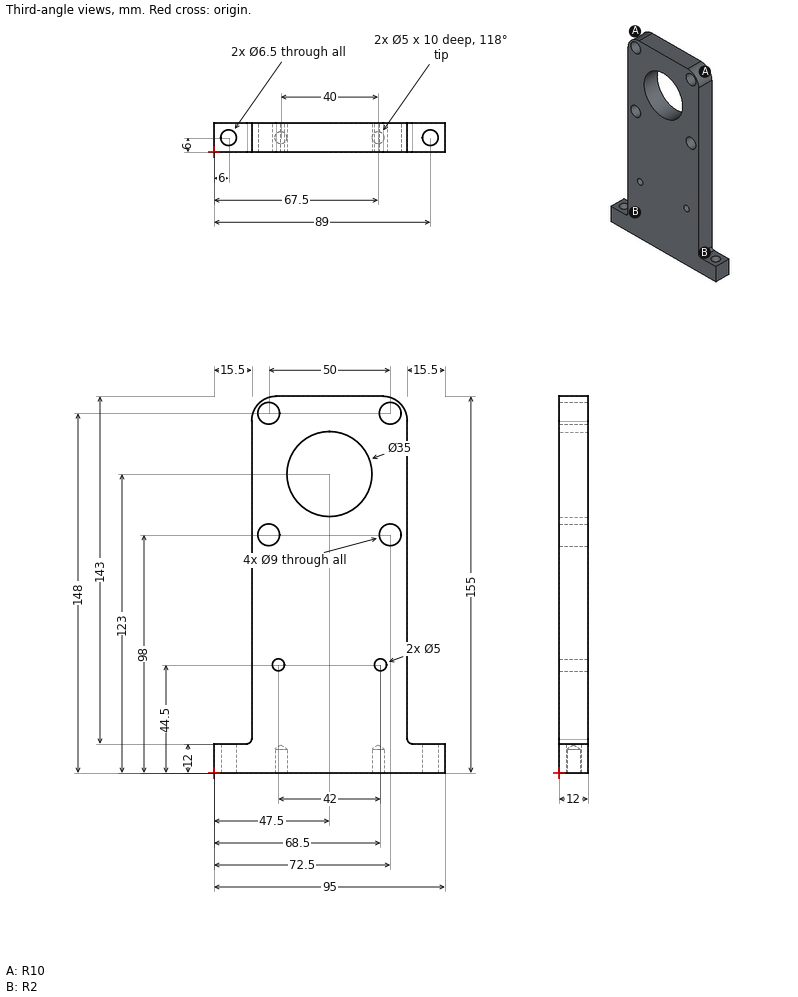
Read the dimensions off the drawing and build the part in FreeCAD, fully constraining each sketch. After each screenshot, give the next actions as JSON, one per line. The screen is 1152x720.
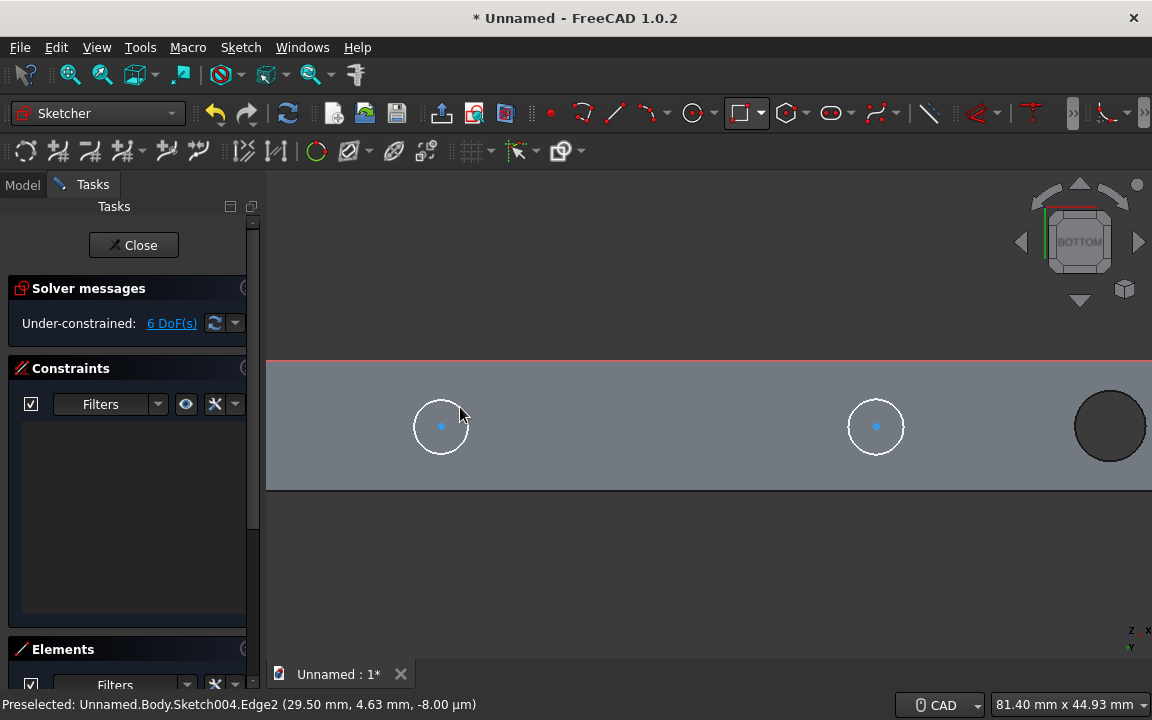
{"action": "left_click", "coordinate": [895, 407]}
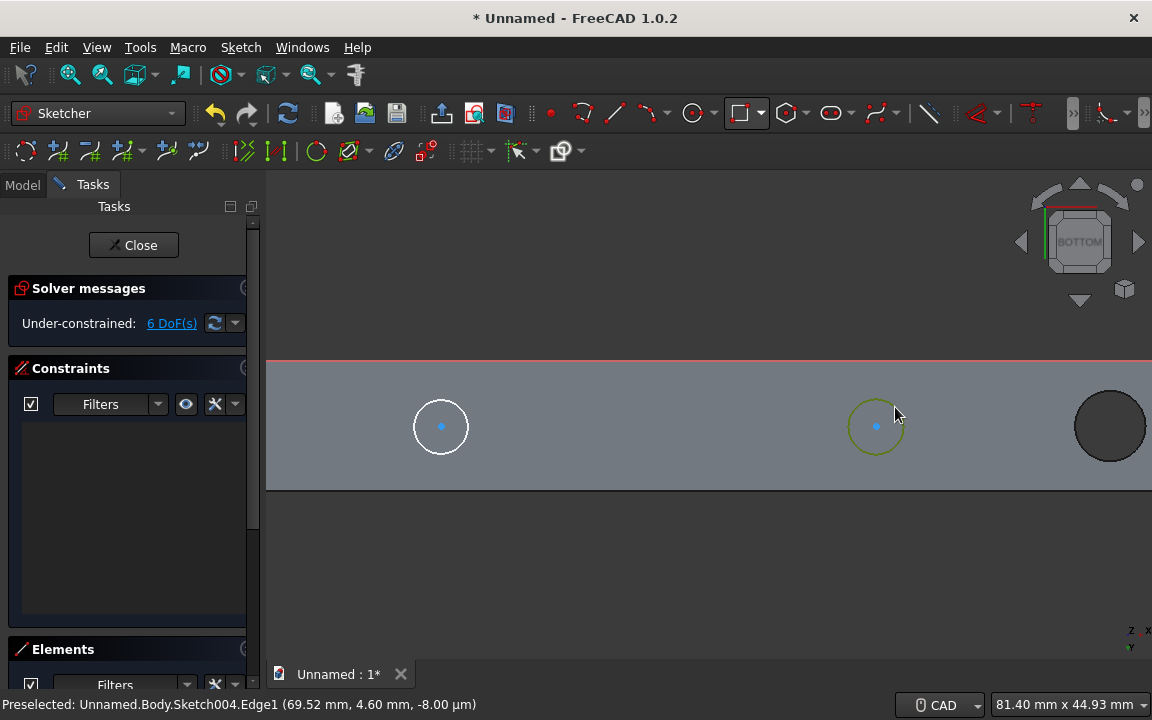
{"action": "left_click", "coordinate": [460, 408]}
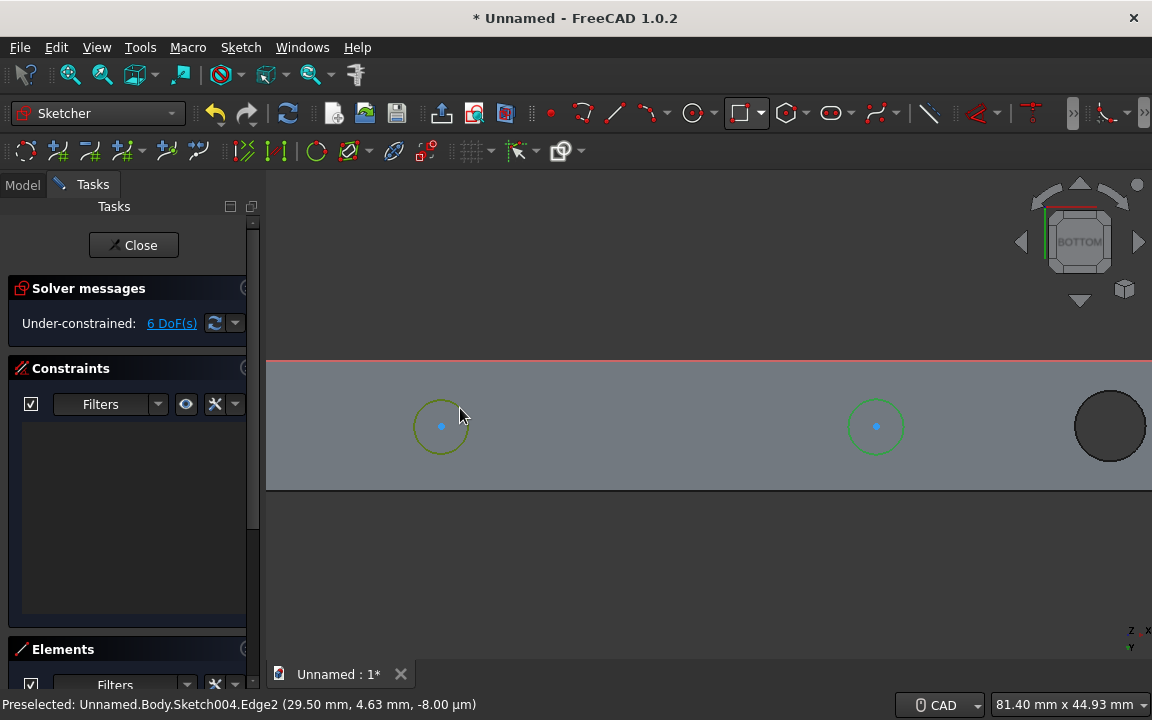
{"action": "key", "text": "e"}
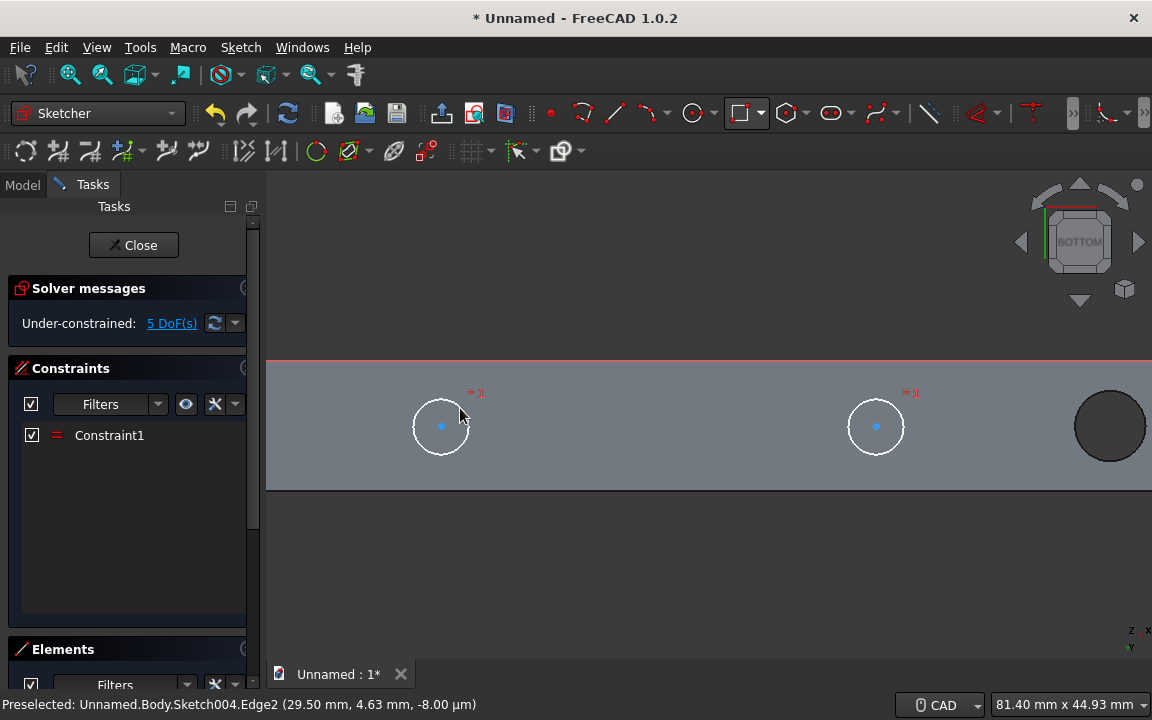
{"action": "left_click", "coordinate": [876, 427]}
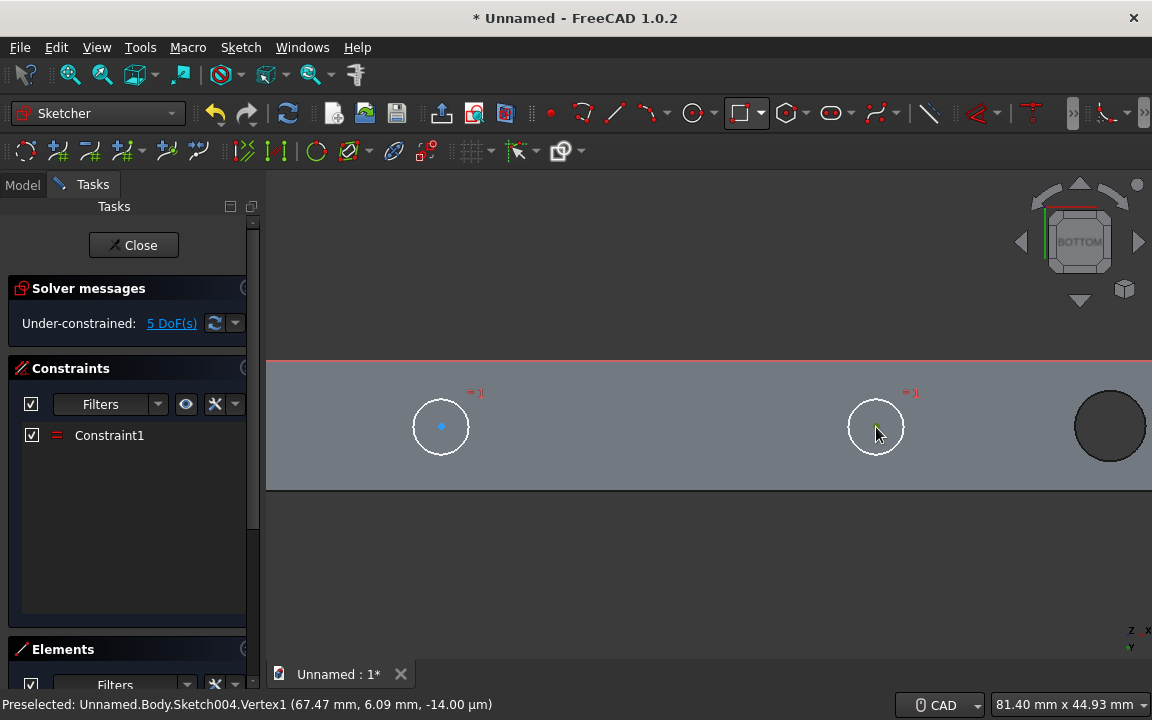
{"action": "left_click", "coordinate": [441, 427]}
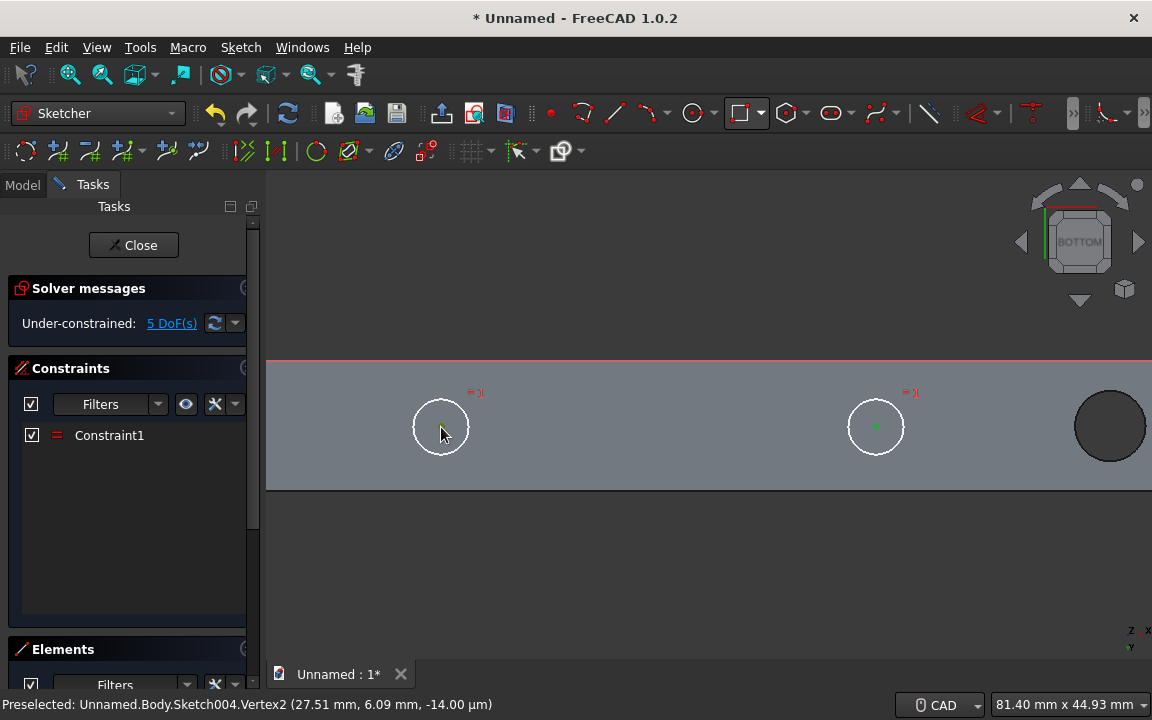
{"action": "key", "text": "h"}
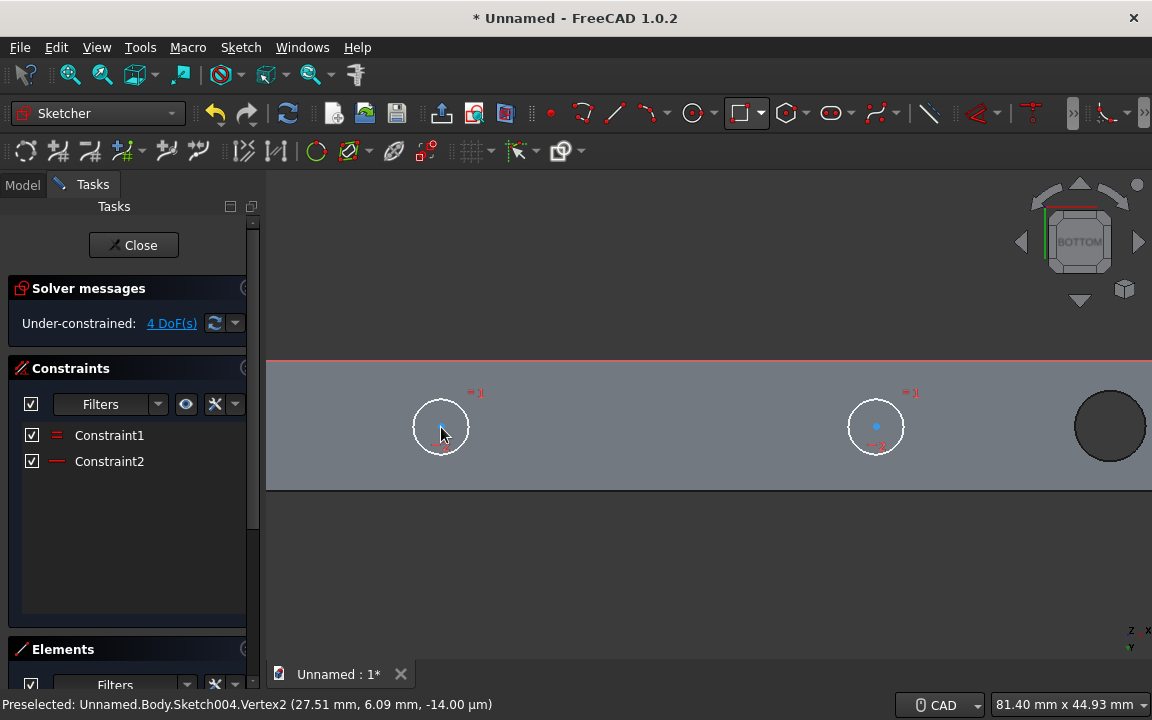
{"action": "left_click", "coordinate": [976, 114]}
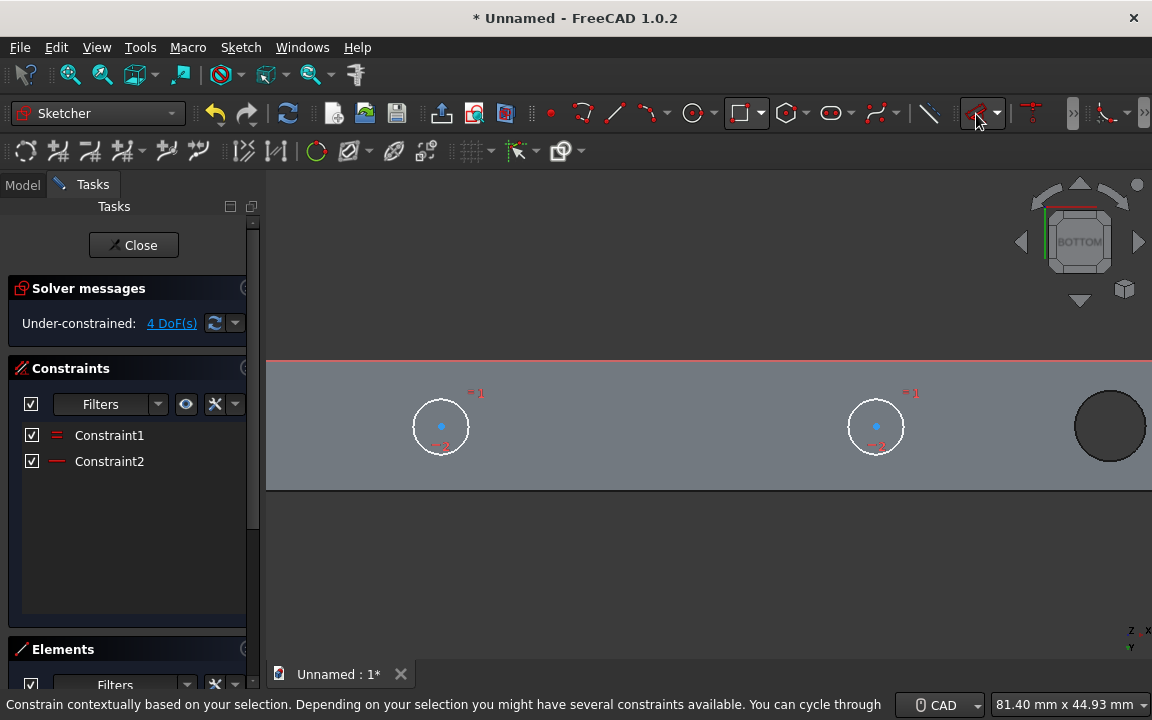
{"action": "left_click", "coordinate": [895, 407]}
{"action": "left_click", "coordinate": [917, 384]}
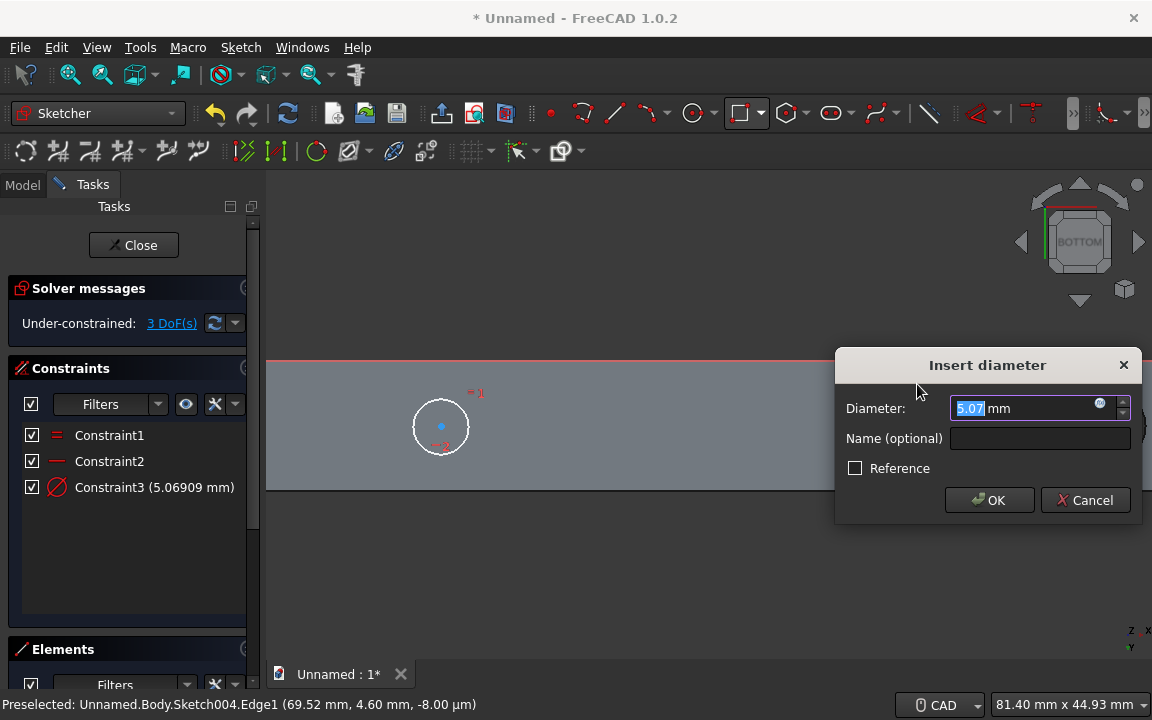
{"action": "type", "text": "5"}
{"action": "key", "text": "Return"}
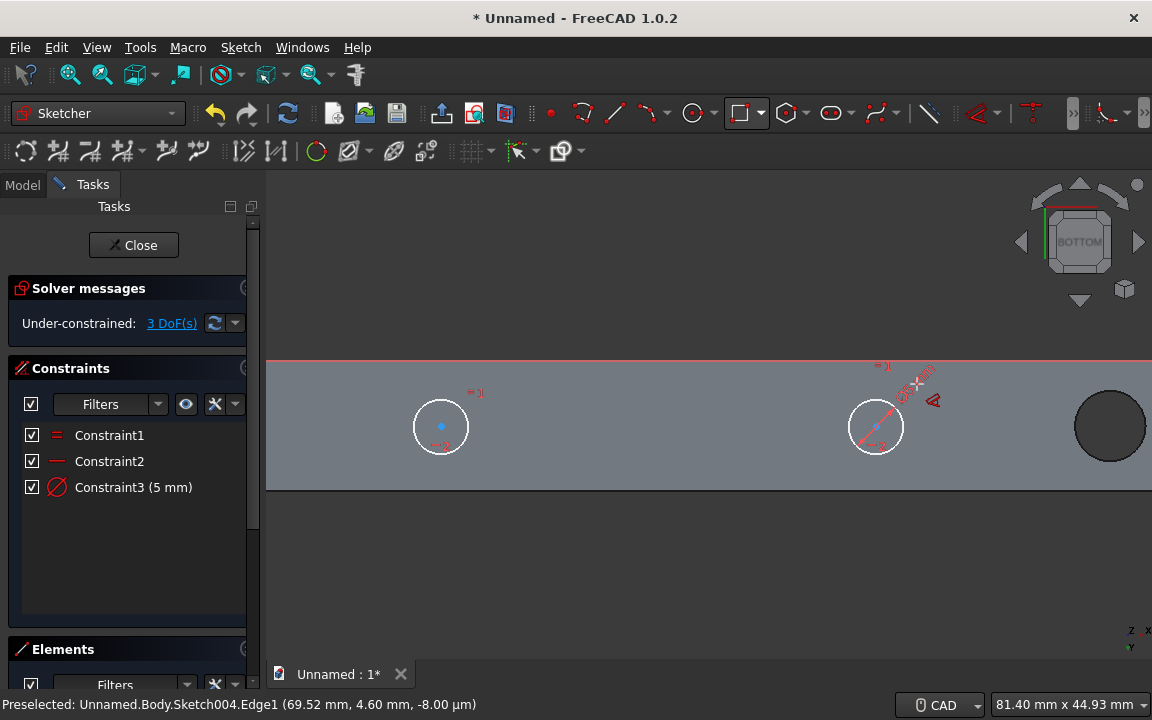
{"action": "left_click", "coordinate": [876, 427]}
{"action": "left_click", "coordinate": [934, 409]}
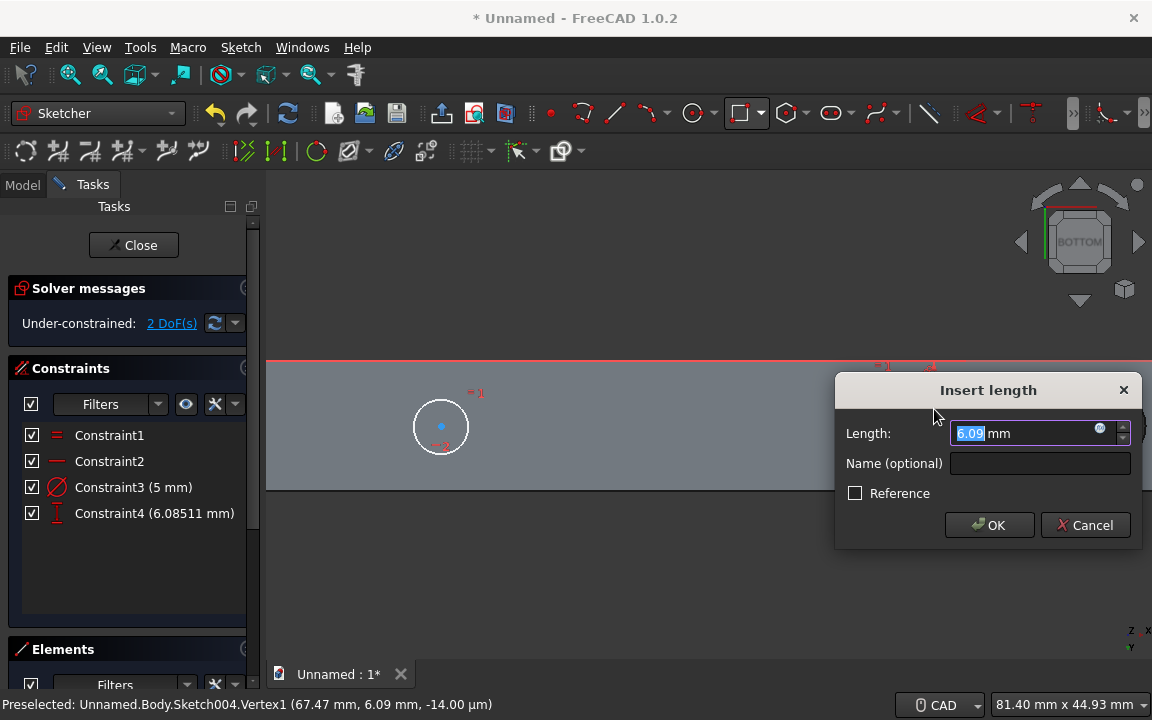
{"action": "type", "text": "6"}
{"action": "key", "text": "Return"}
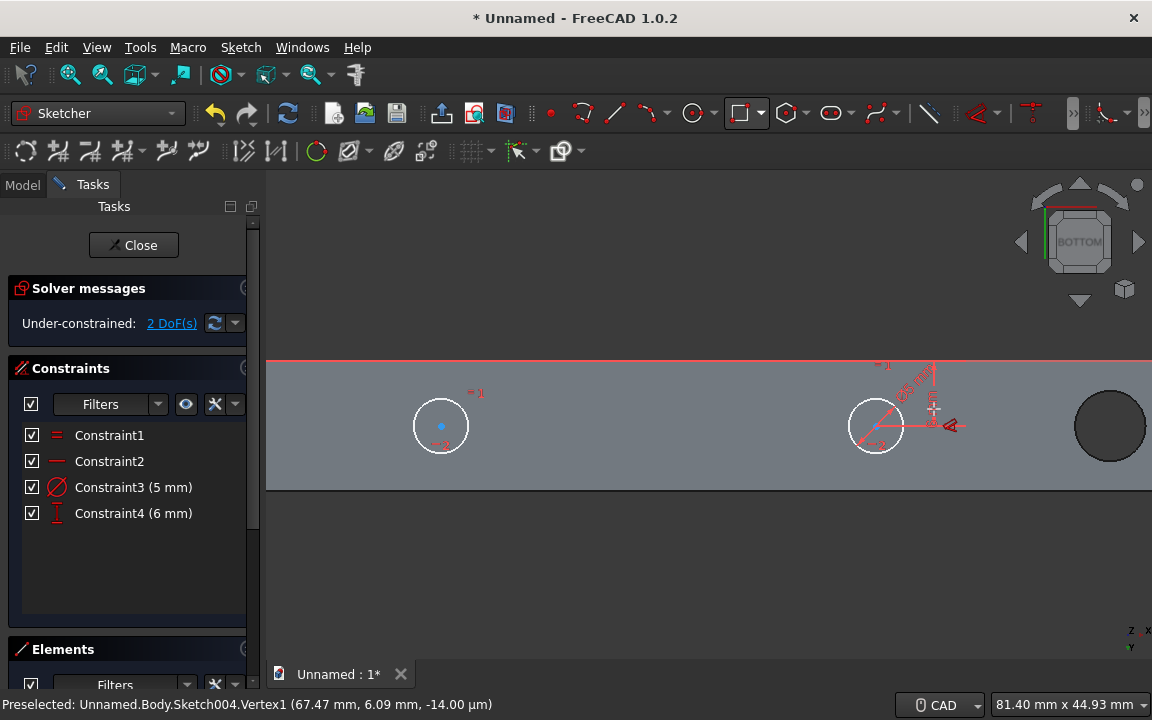
{"action": "left_click", "coordinate": [876, 426]}